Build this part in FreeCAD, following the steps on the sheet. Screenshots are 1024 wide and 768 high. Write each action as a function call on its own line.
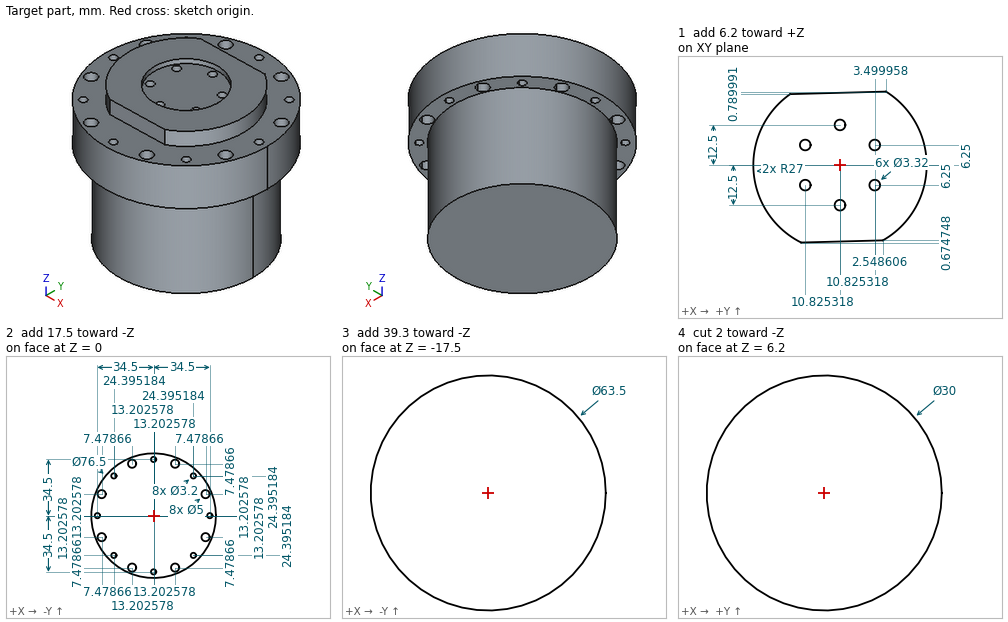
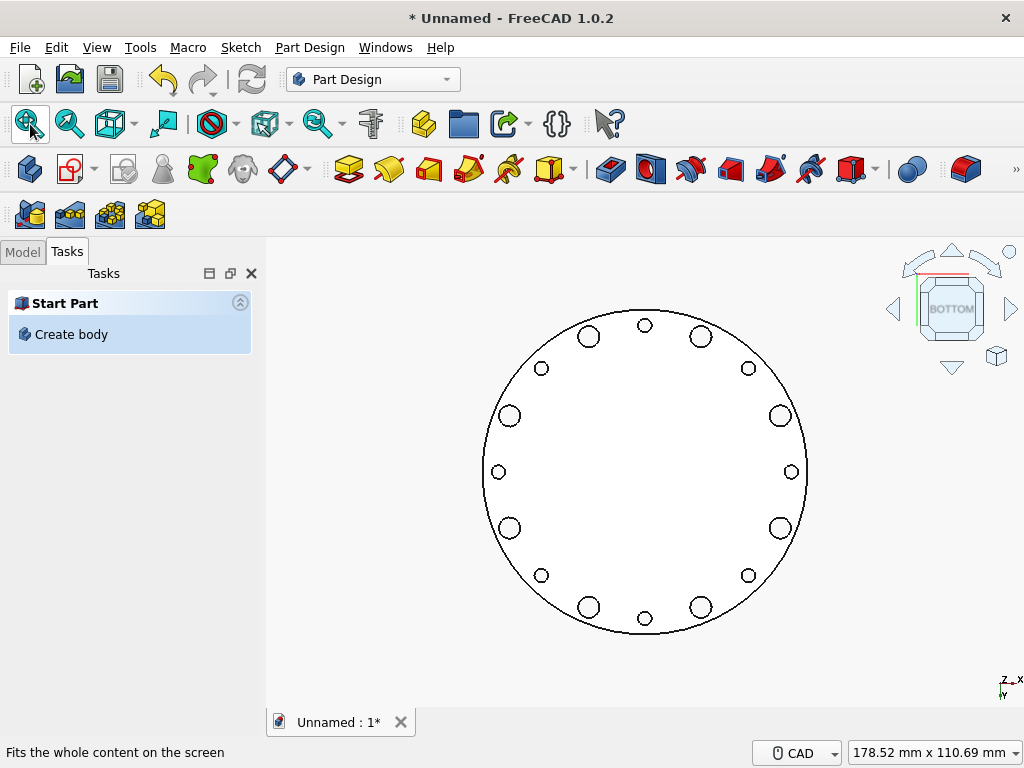
click(645, 471)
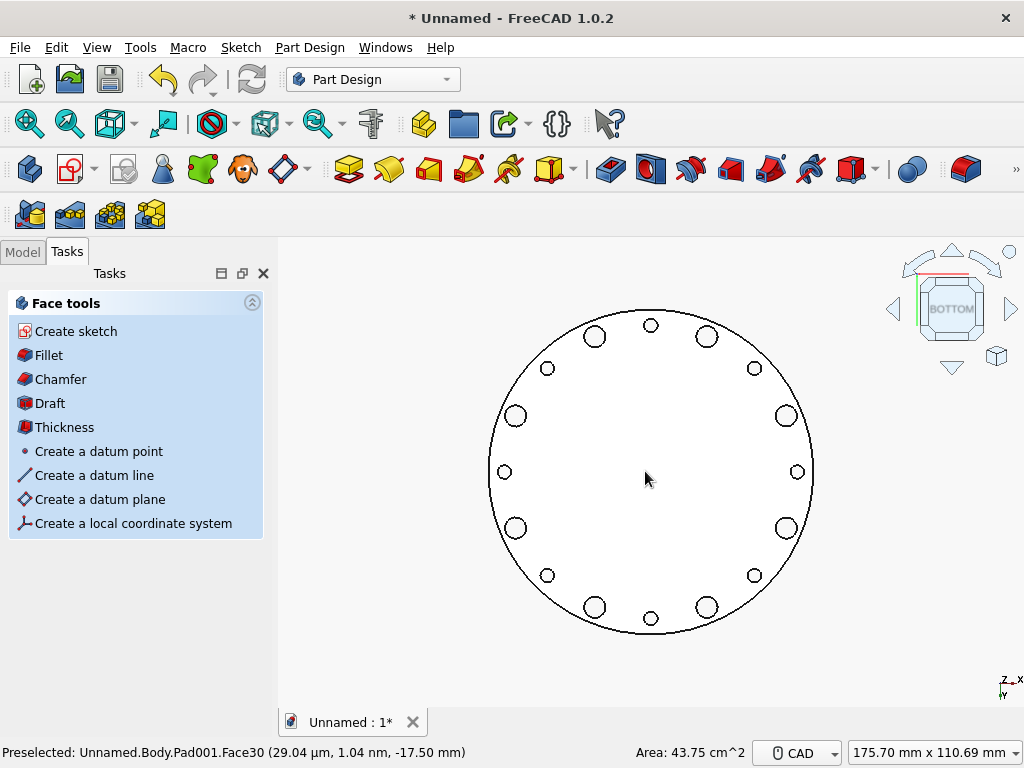
click(70, 170)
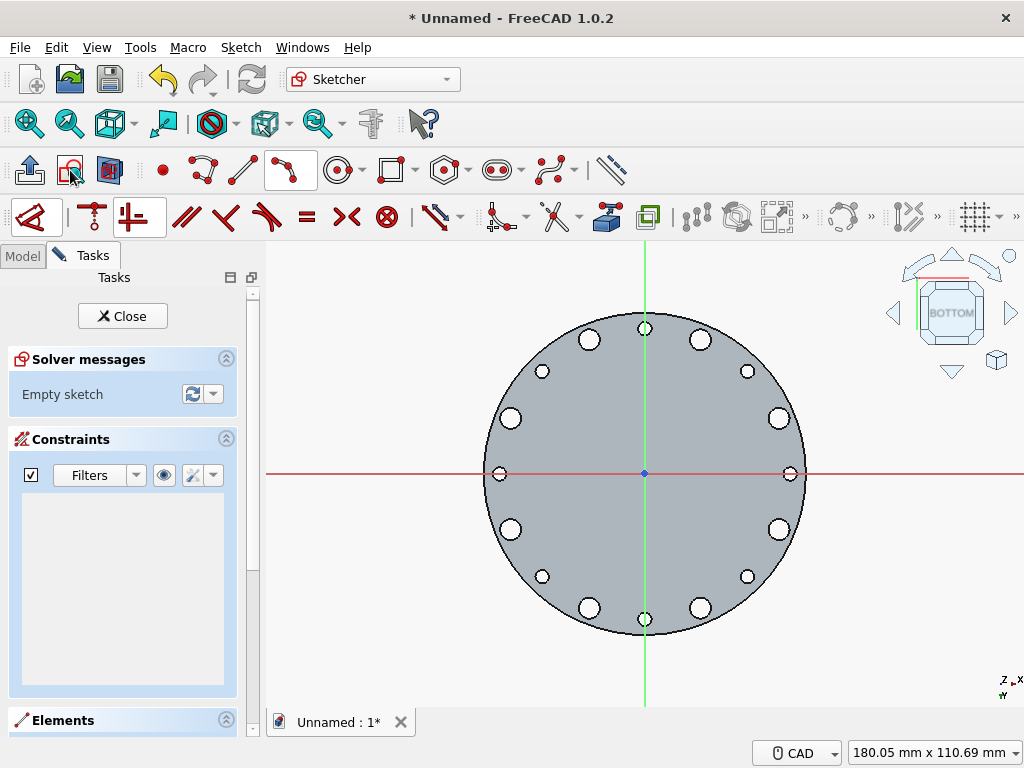
key(g)
key(c)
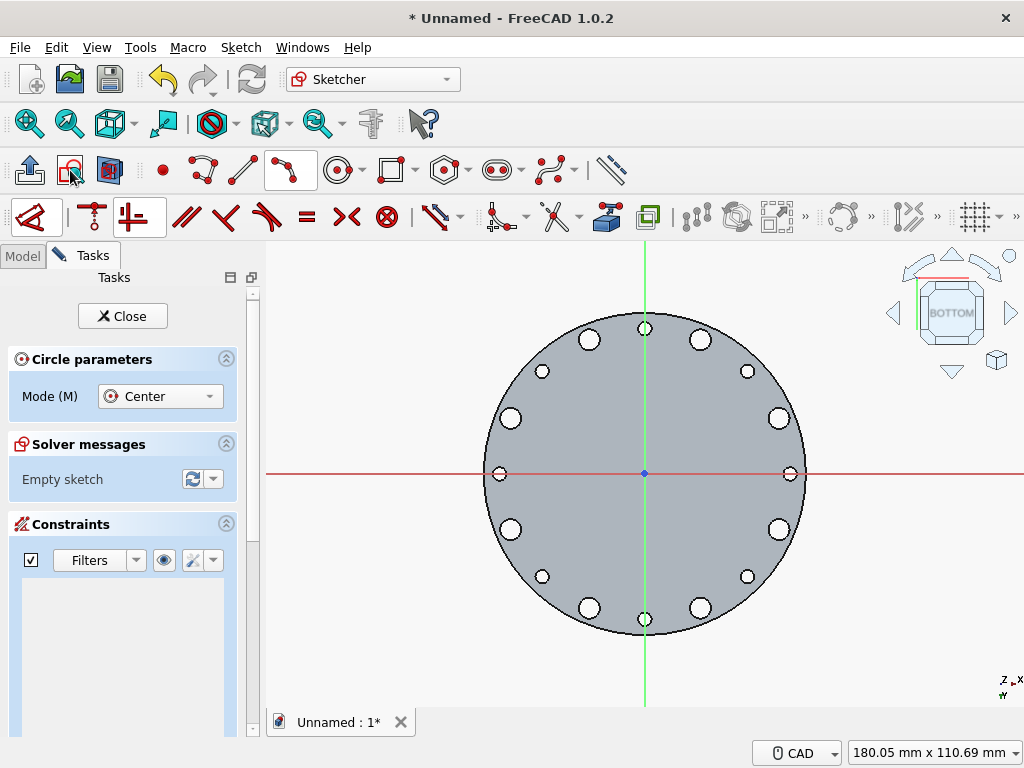
click(645, 474)
move(739, 379)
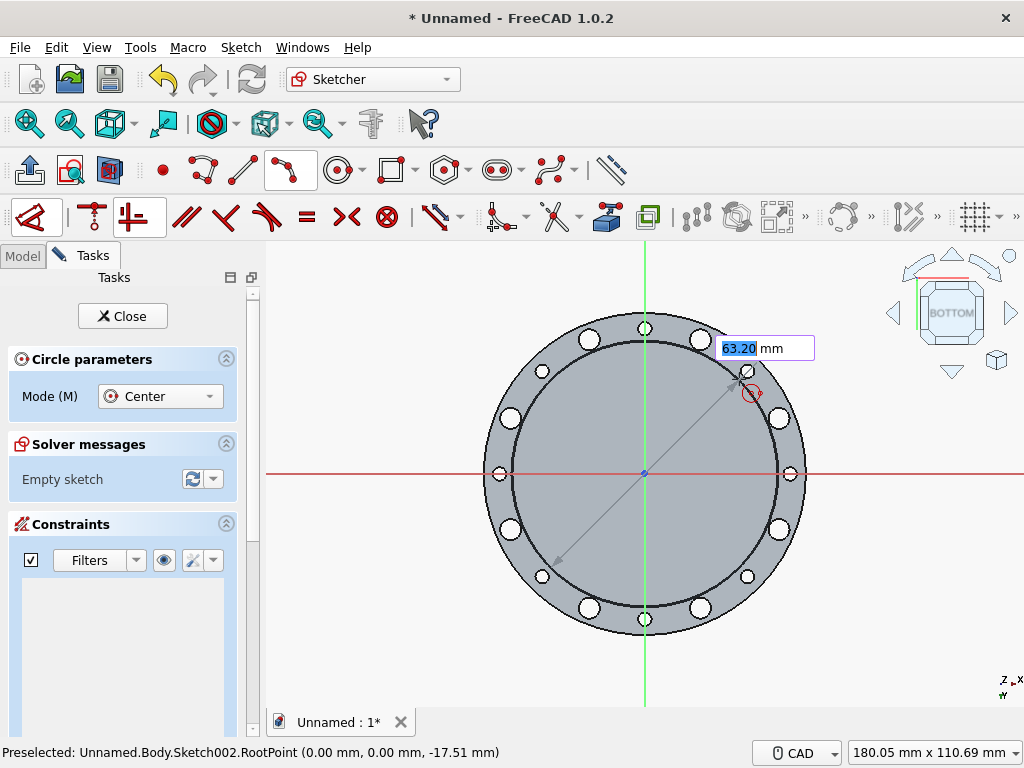
text(63.5)
key(Return)
key(Escape)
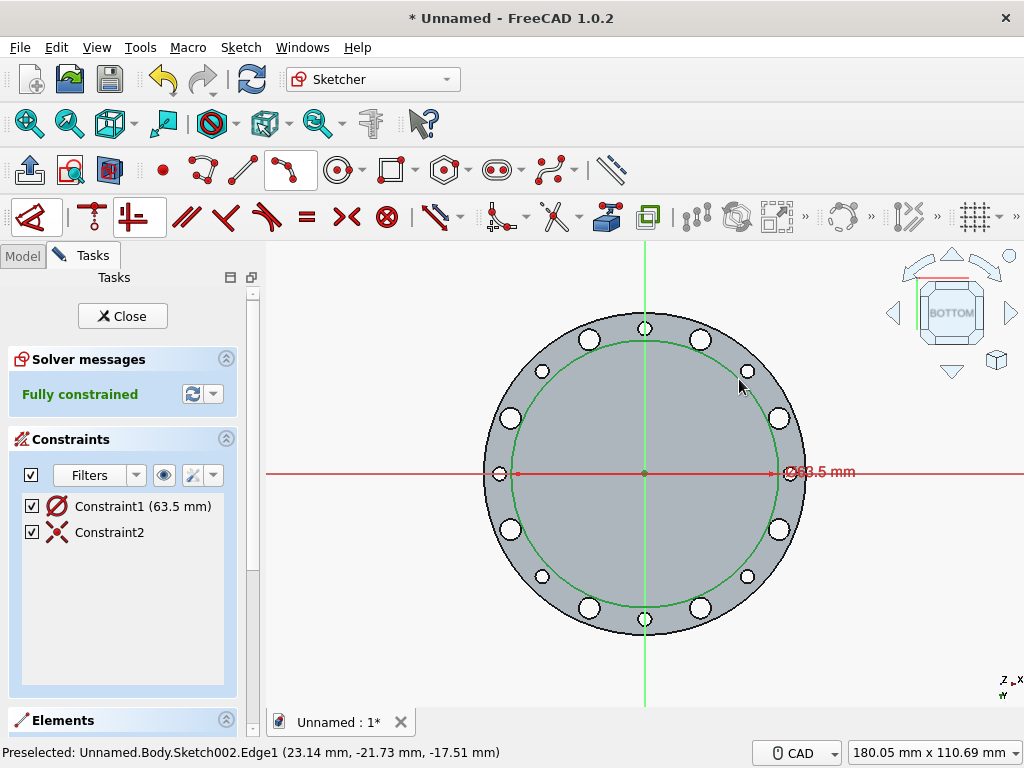
click(123, 316)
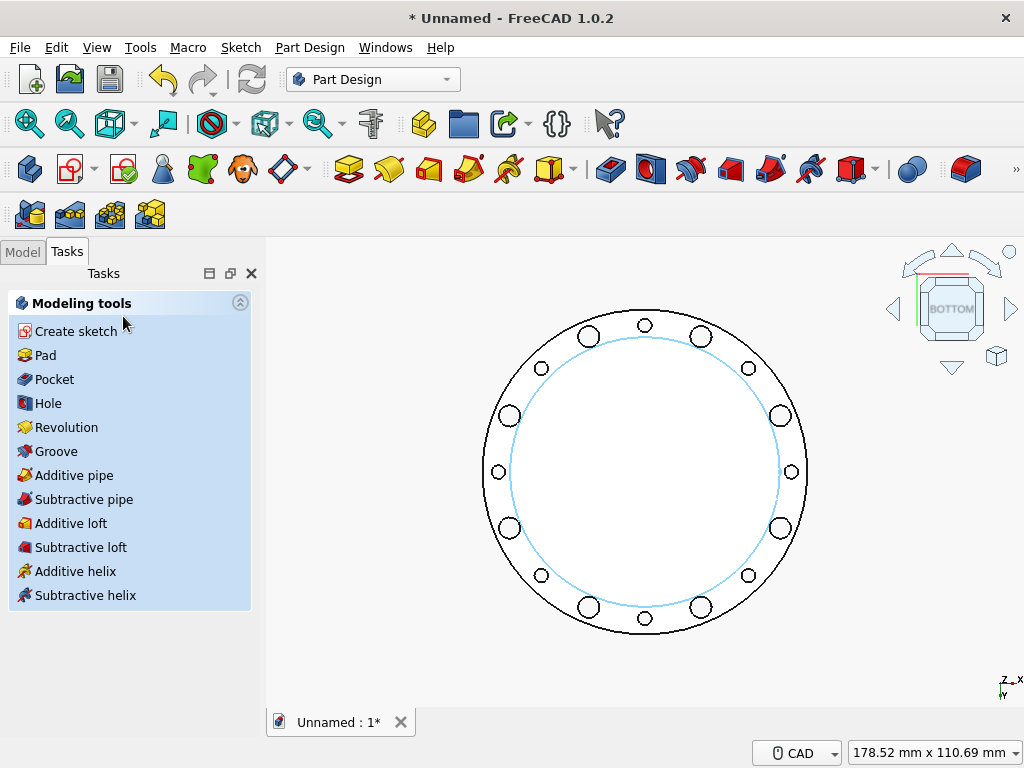
click(350, 170)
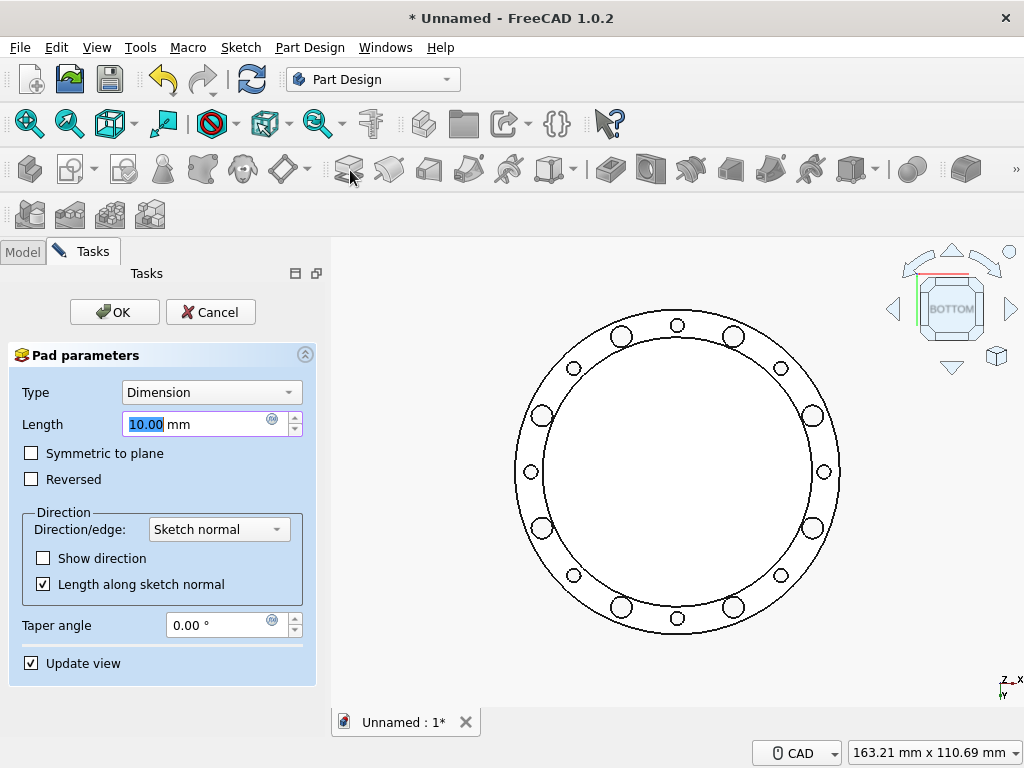
text(39.3)
key(Tab)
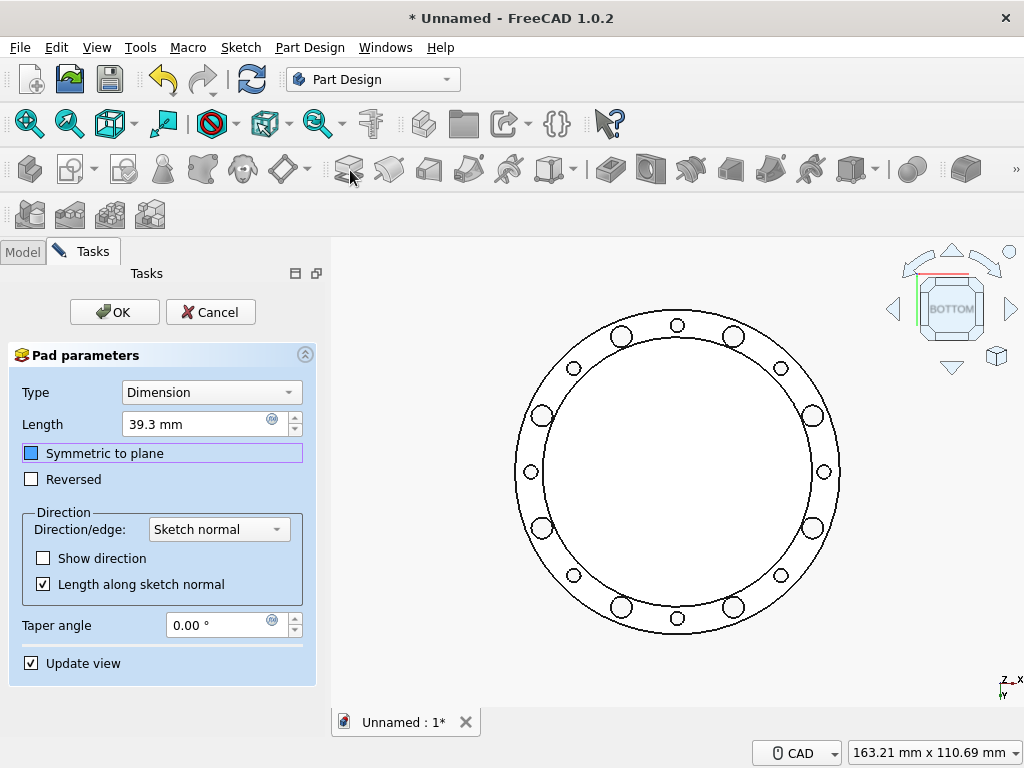
click(115, 312)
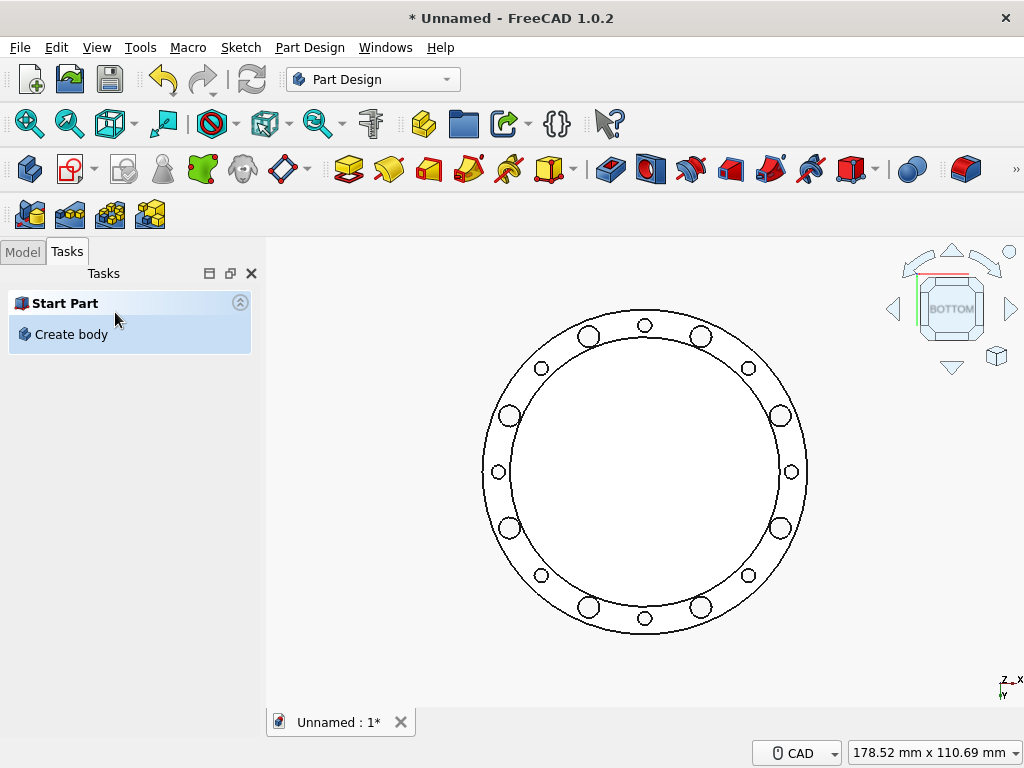
key(0)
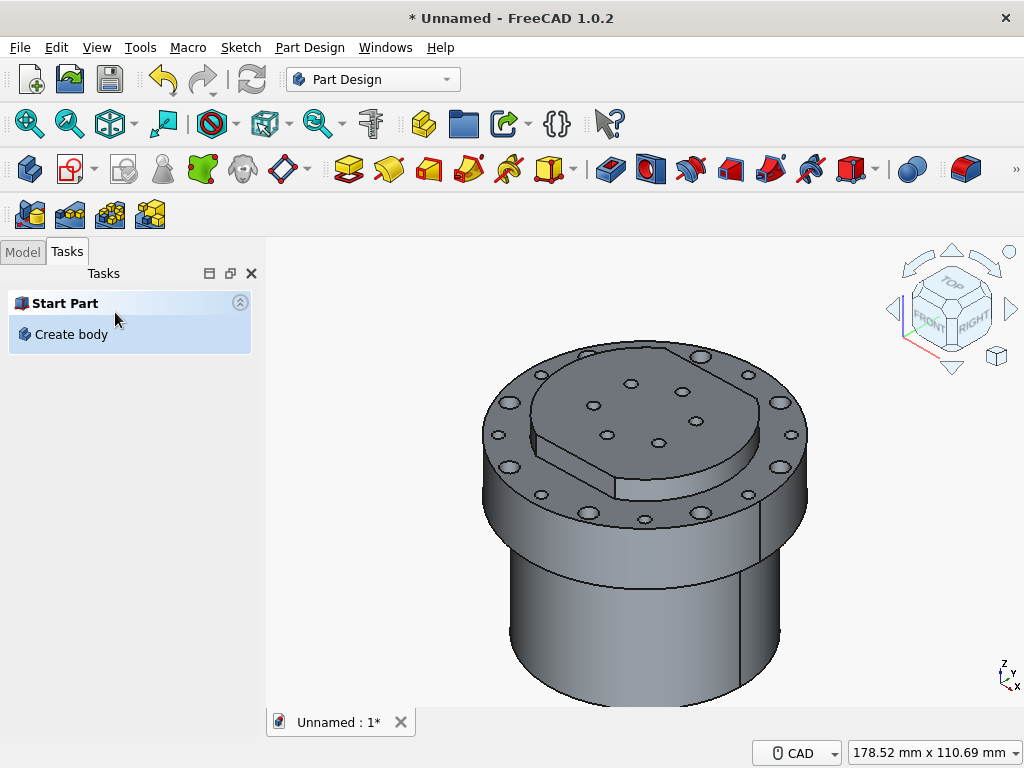
key(v)
key(f)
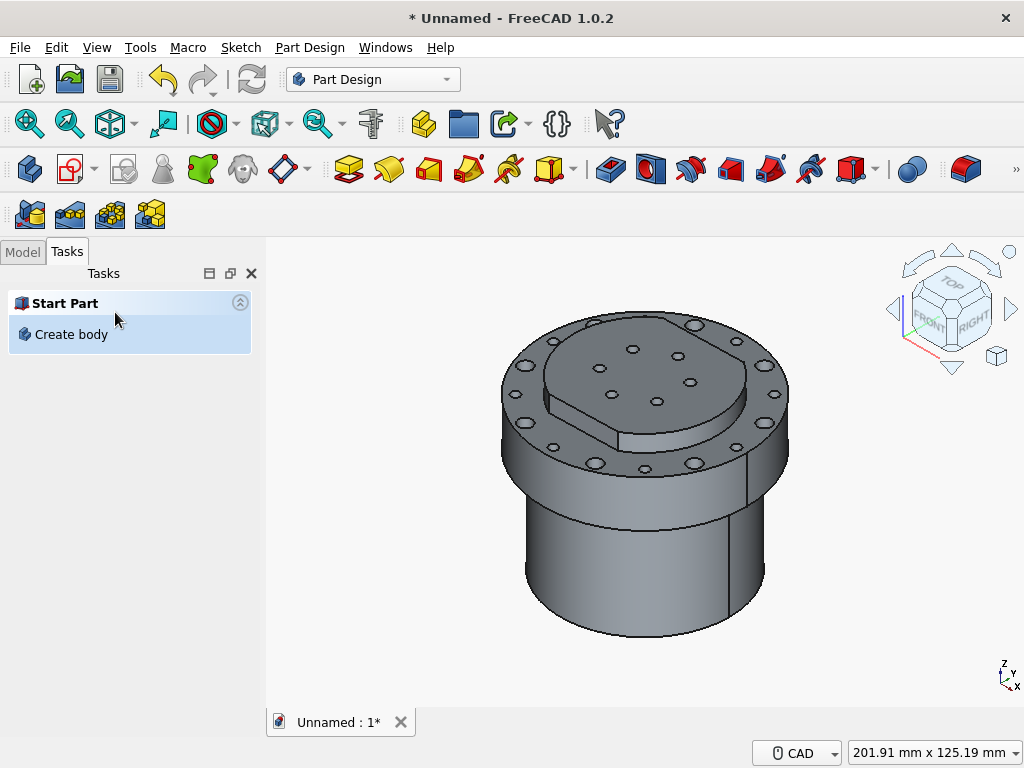
click(643, 375)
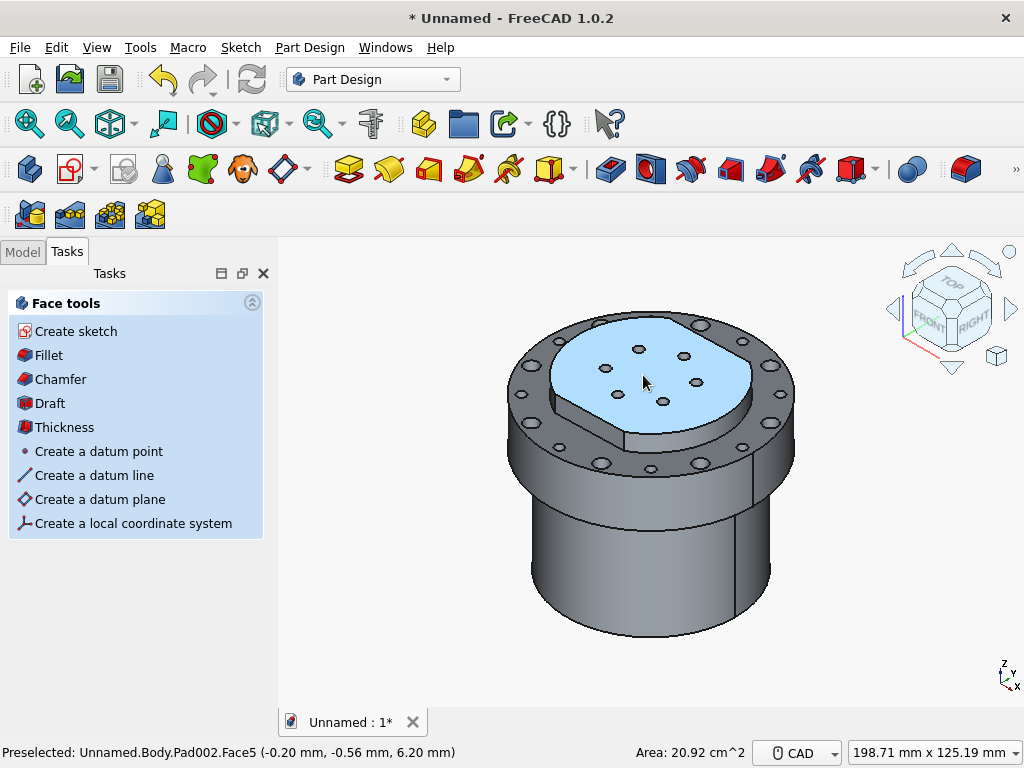
click(70, 170)